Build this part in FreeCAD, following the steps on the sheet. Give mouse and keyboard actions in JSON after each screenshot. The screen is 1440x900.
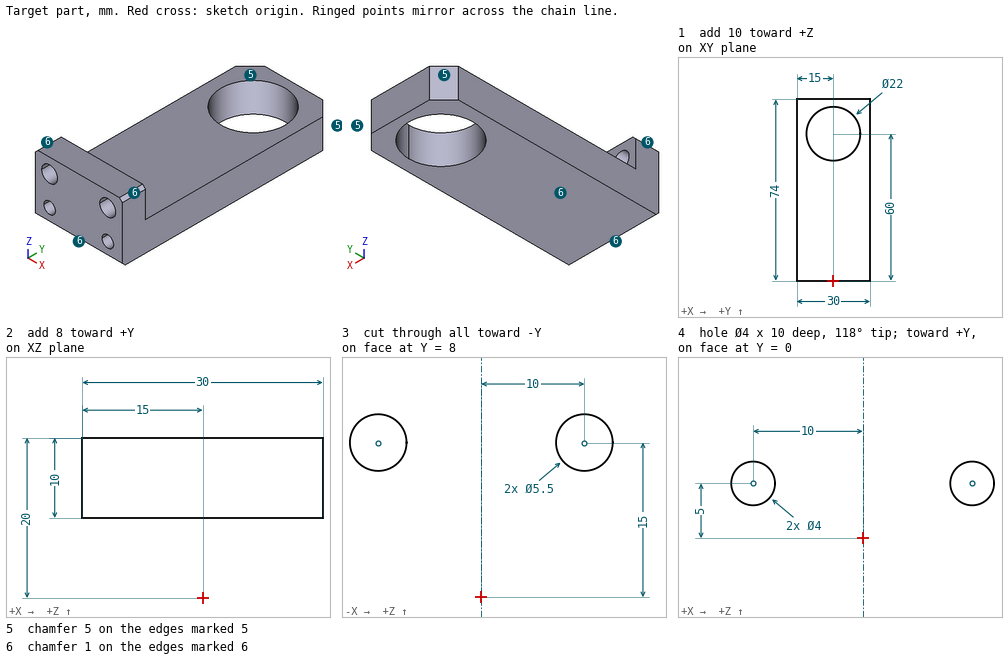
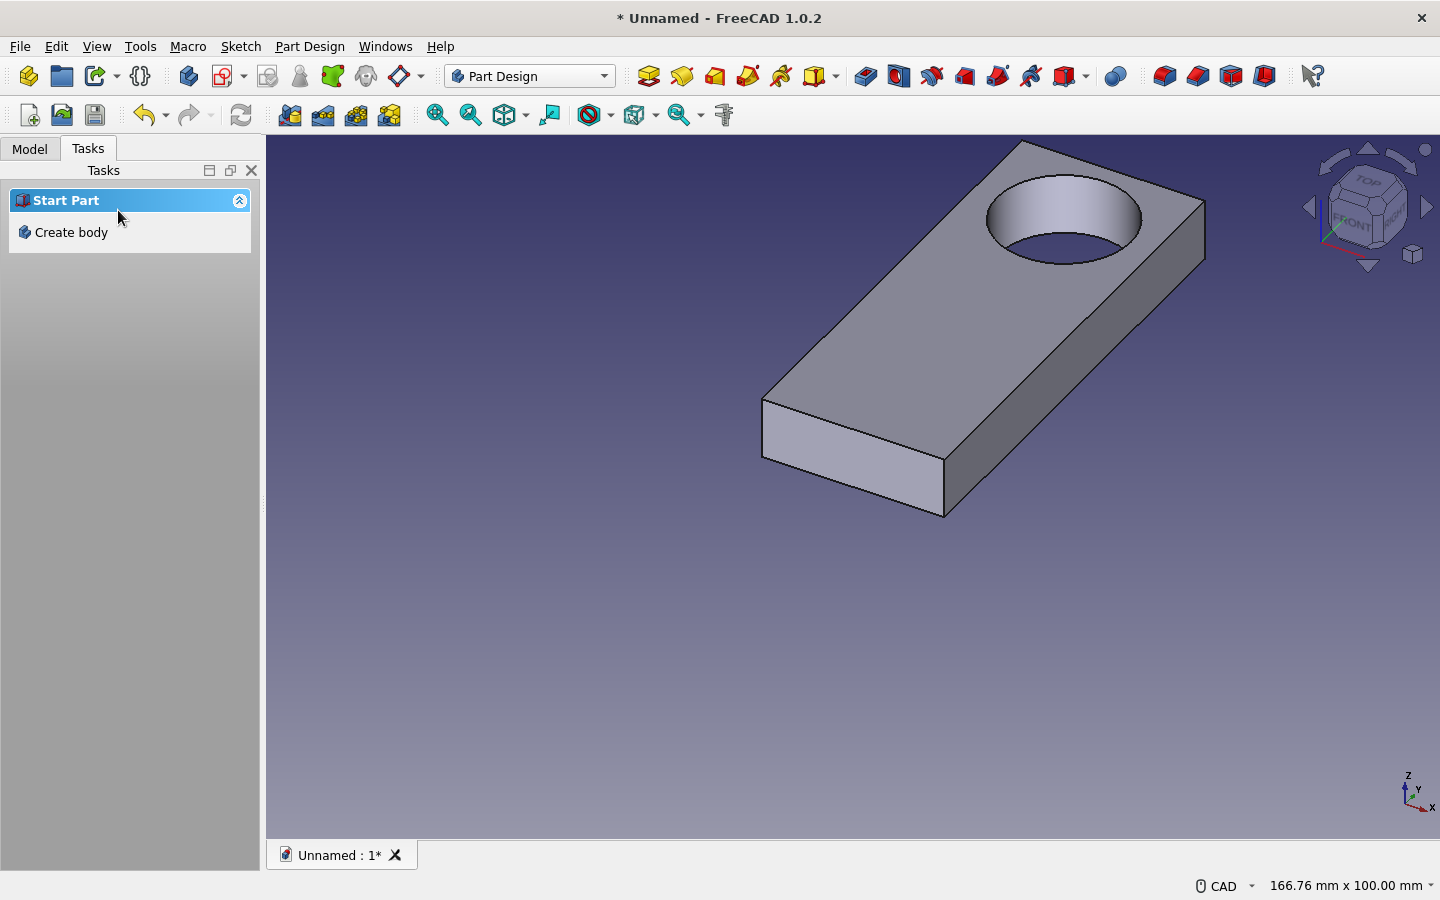
{"action": "left_click", "coordinate": [222, 76]}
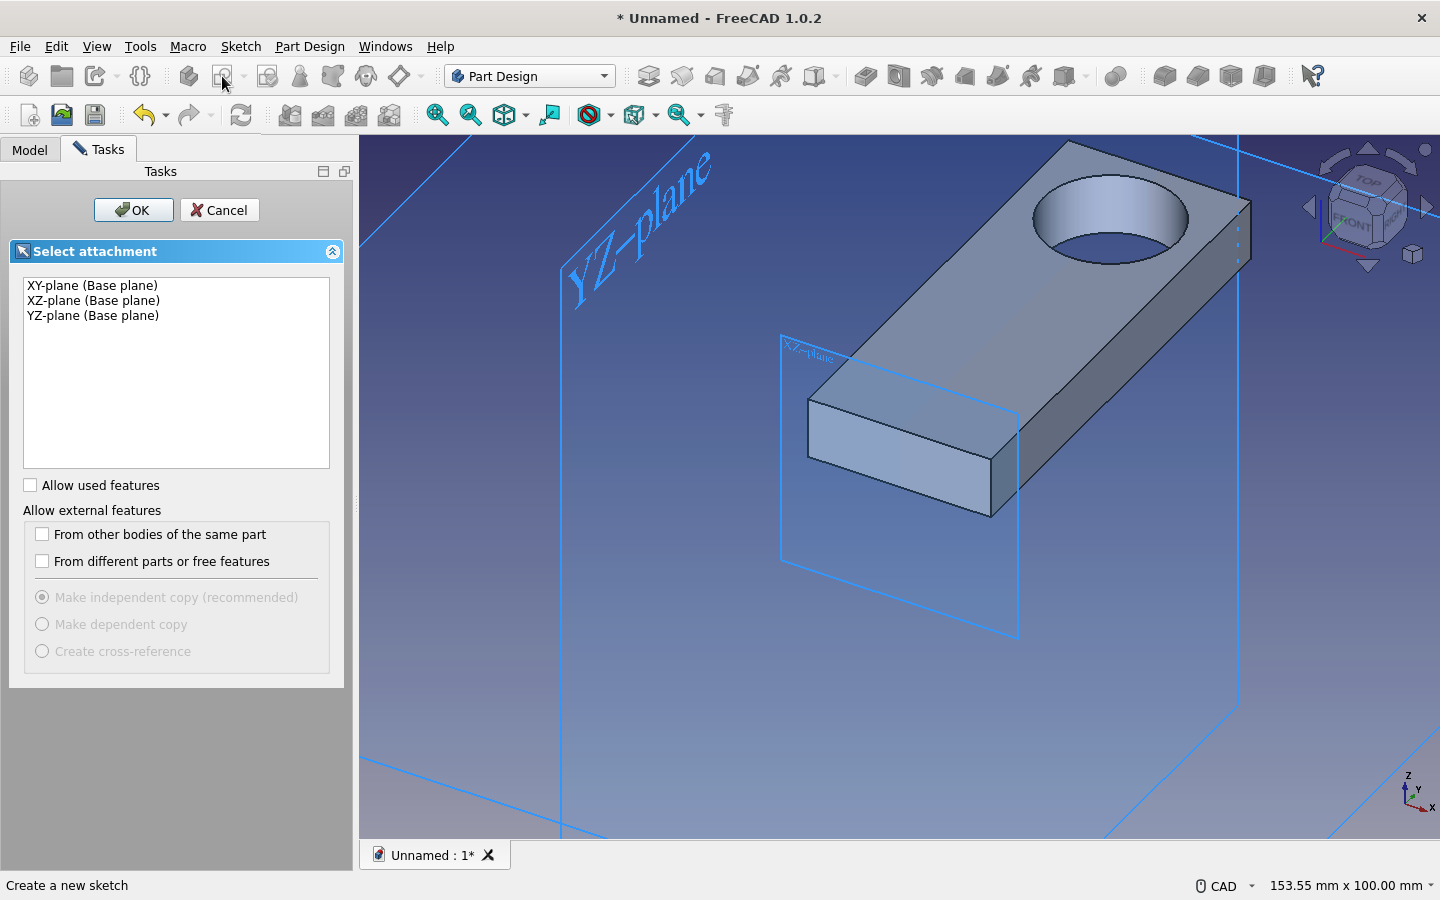
{"action": "left_click", "coordinate": [84, 300]}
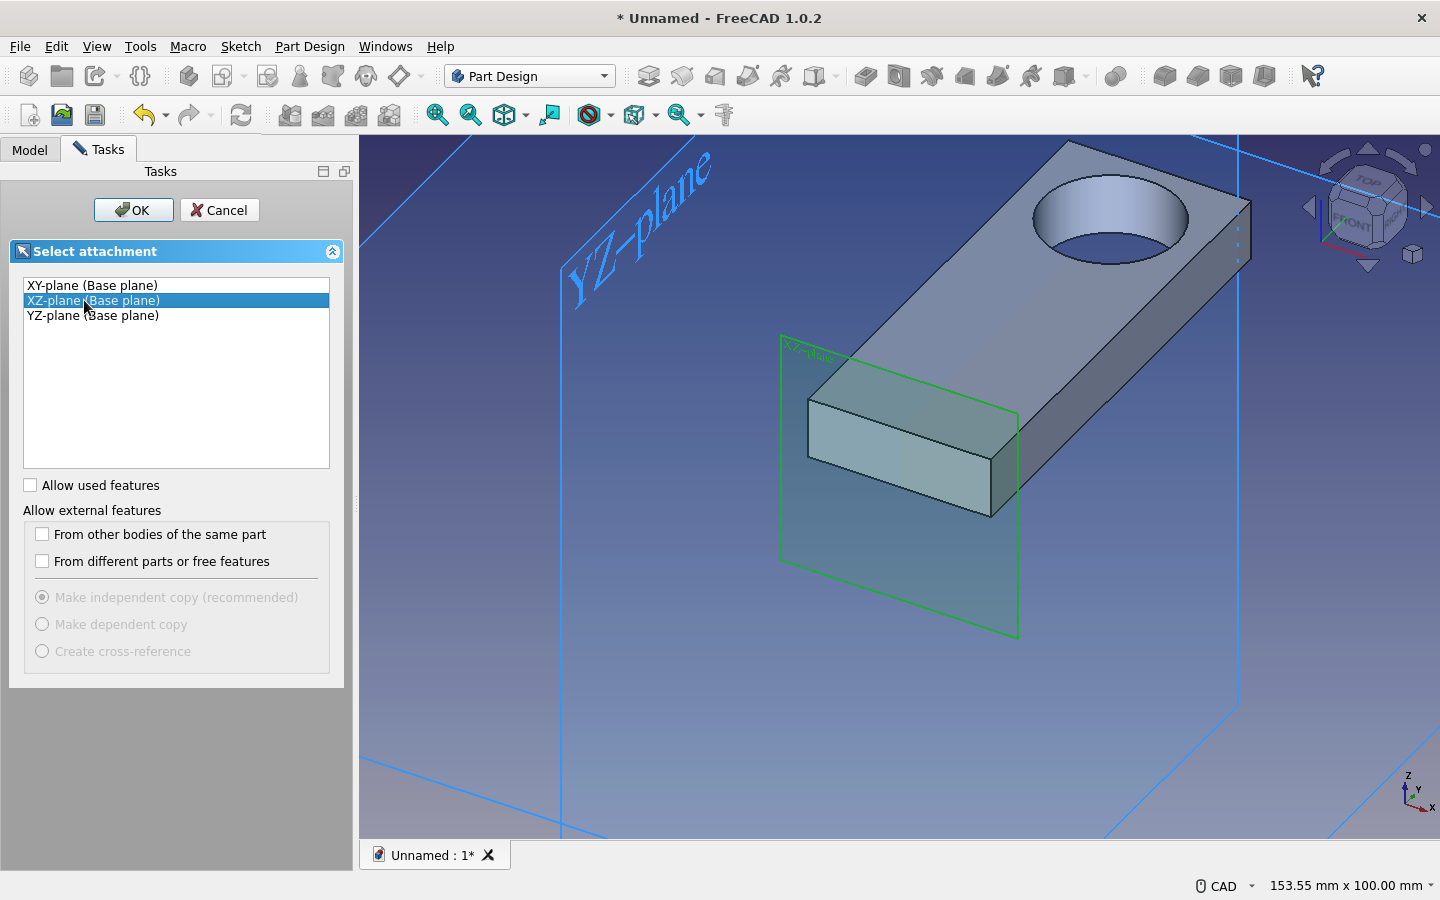
{"action": "left_click", "coordinate": [134, 210]}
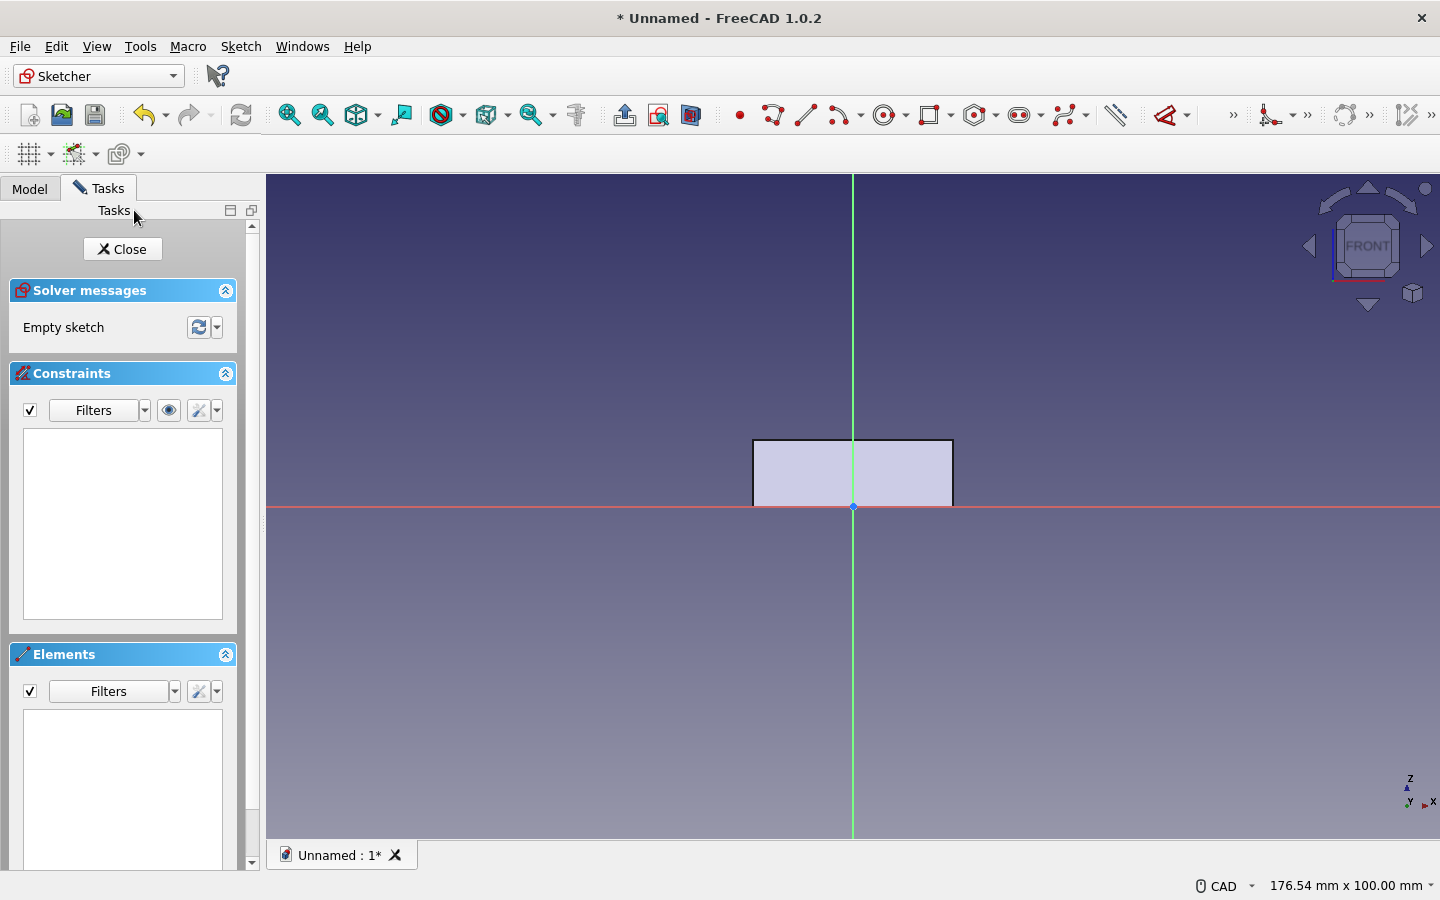
{"action": "scroll", "coordinate": [883, 411], "scroll_direction": "up", "scroll_amount": 6}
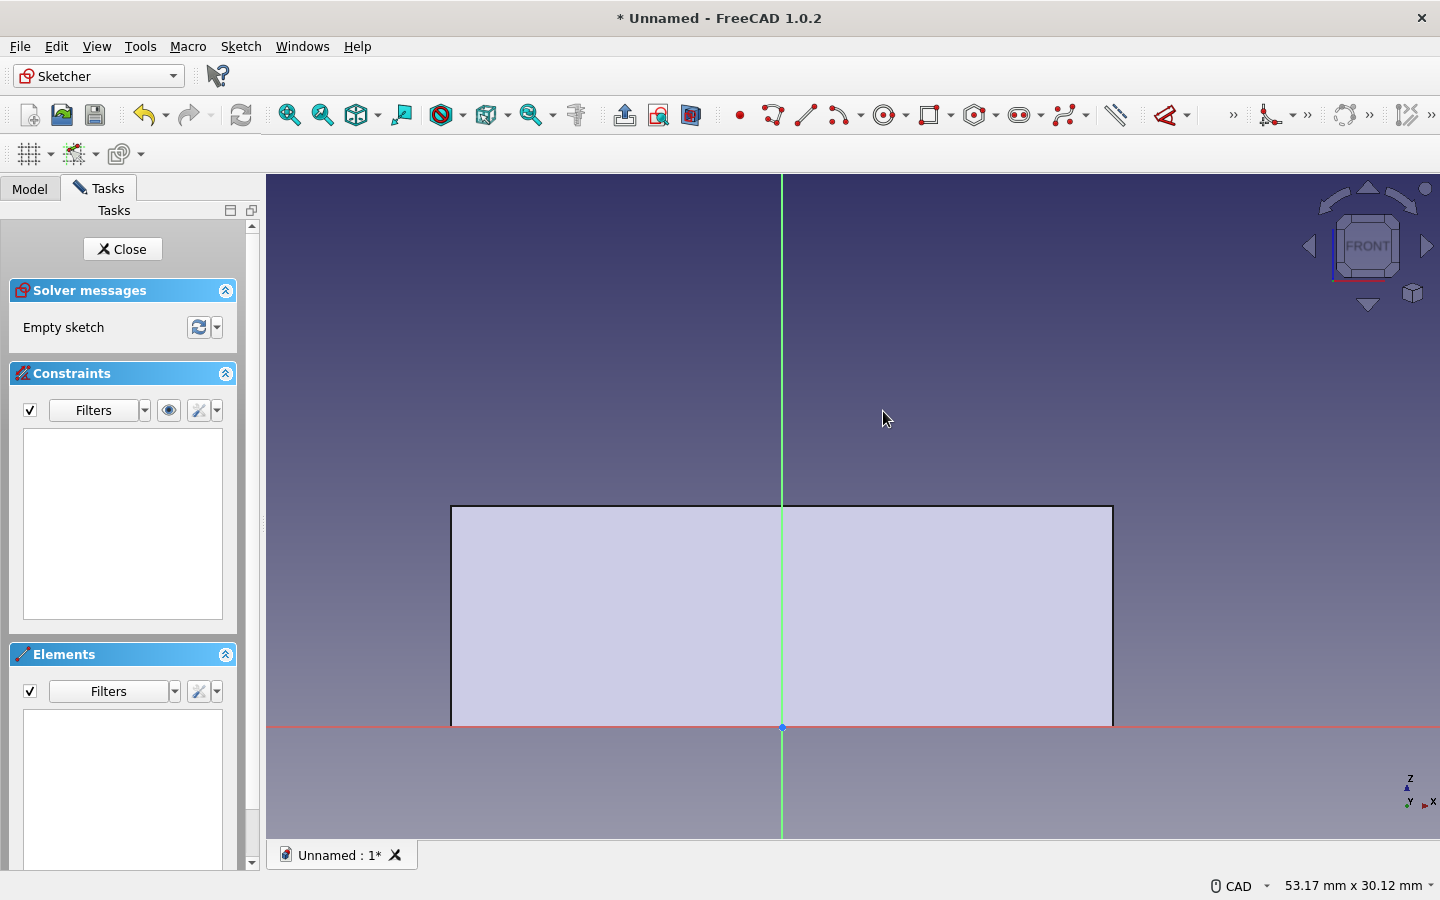
{"action": "left_click", "coordinate": [928, 116]}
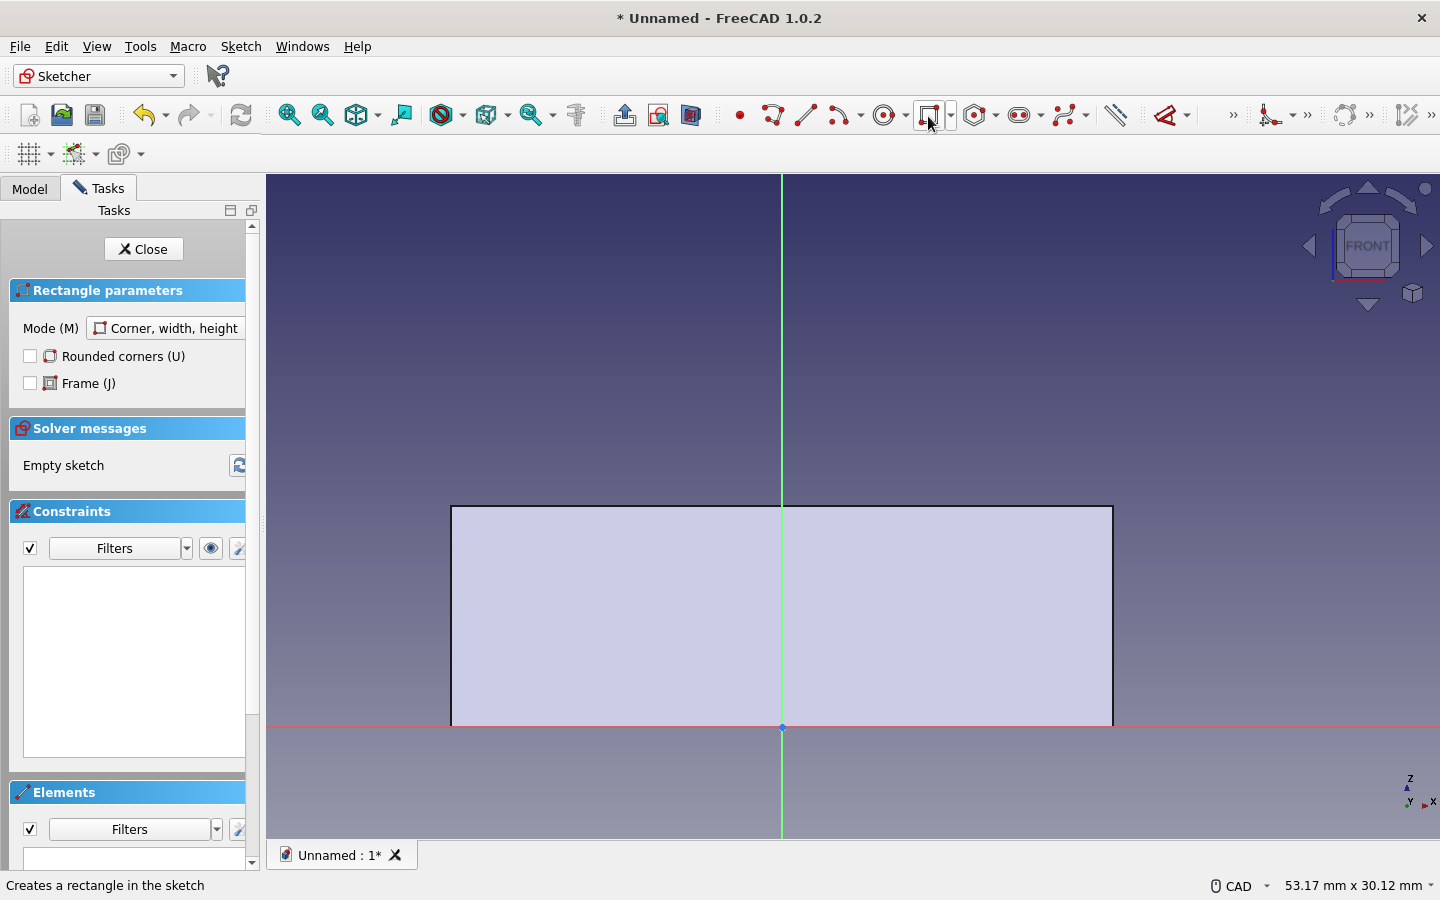
{"action": "left_click", "coordinate": [451, 286]}
{"action": "left_click", "coordinate": [1113, 506]}
{"action": "key", "text": "Escape"}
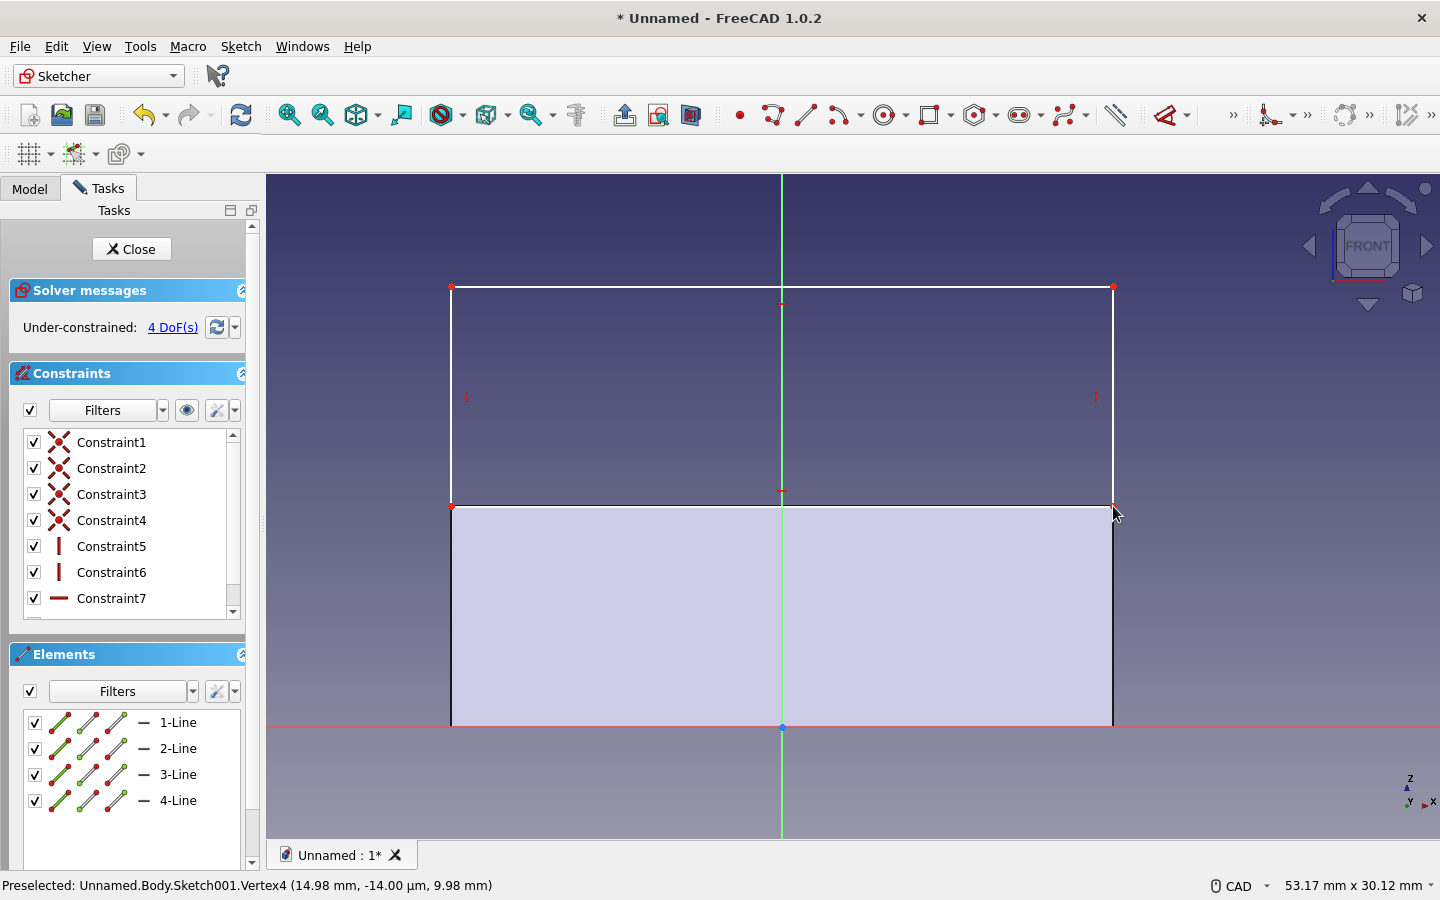
{"action": "left_click", "coordinate": [1164, 116]}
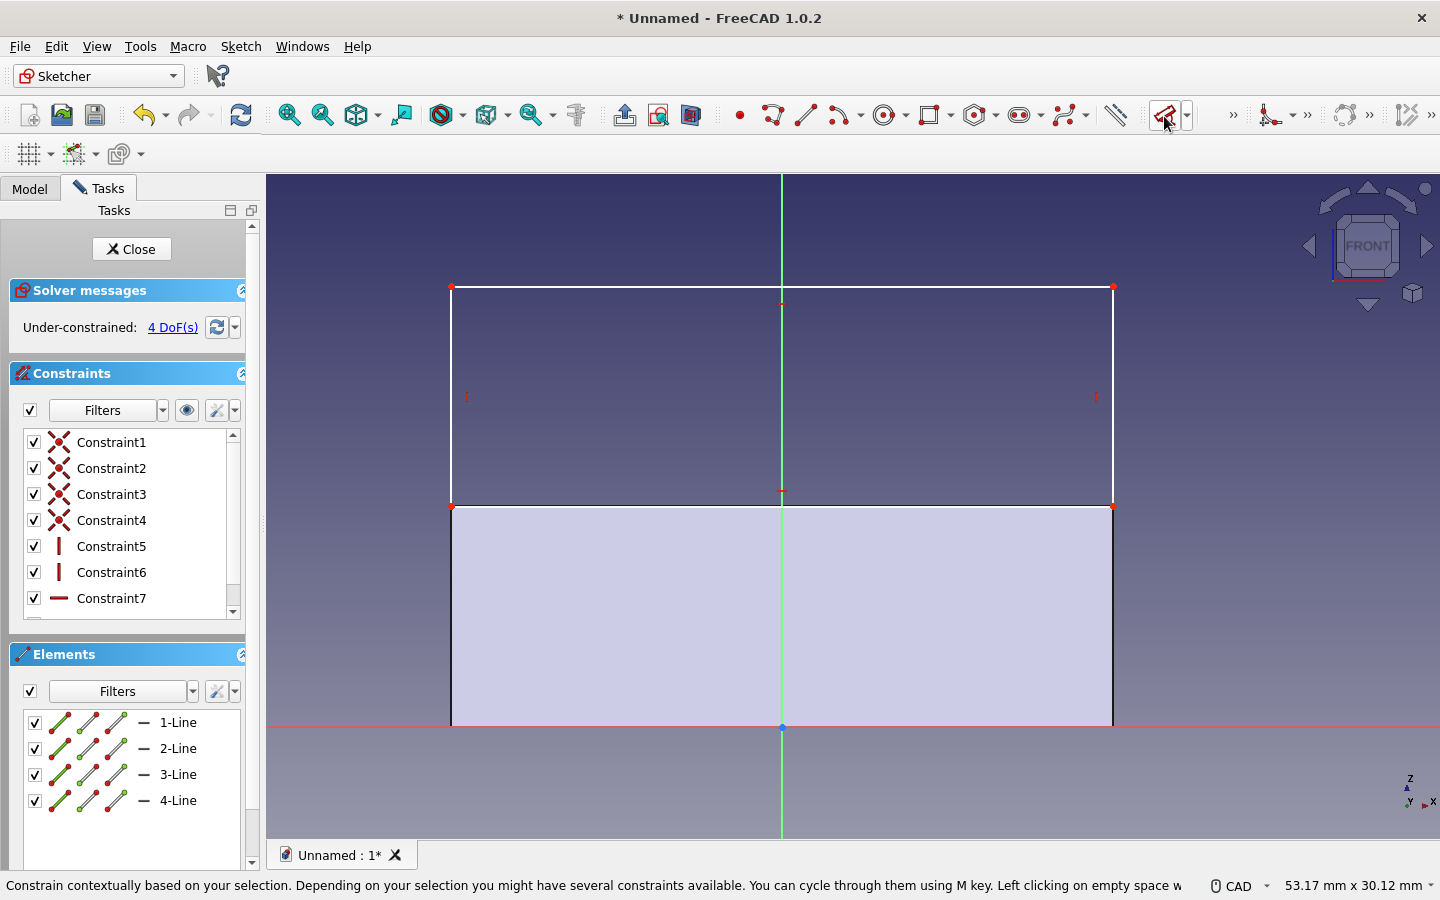
{"action": "left_click", "coordinate": [451, 353]}
{"action": "left_click", "coordinate": [417, 397]}